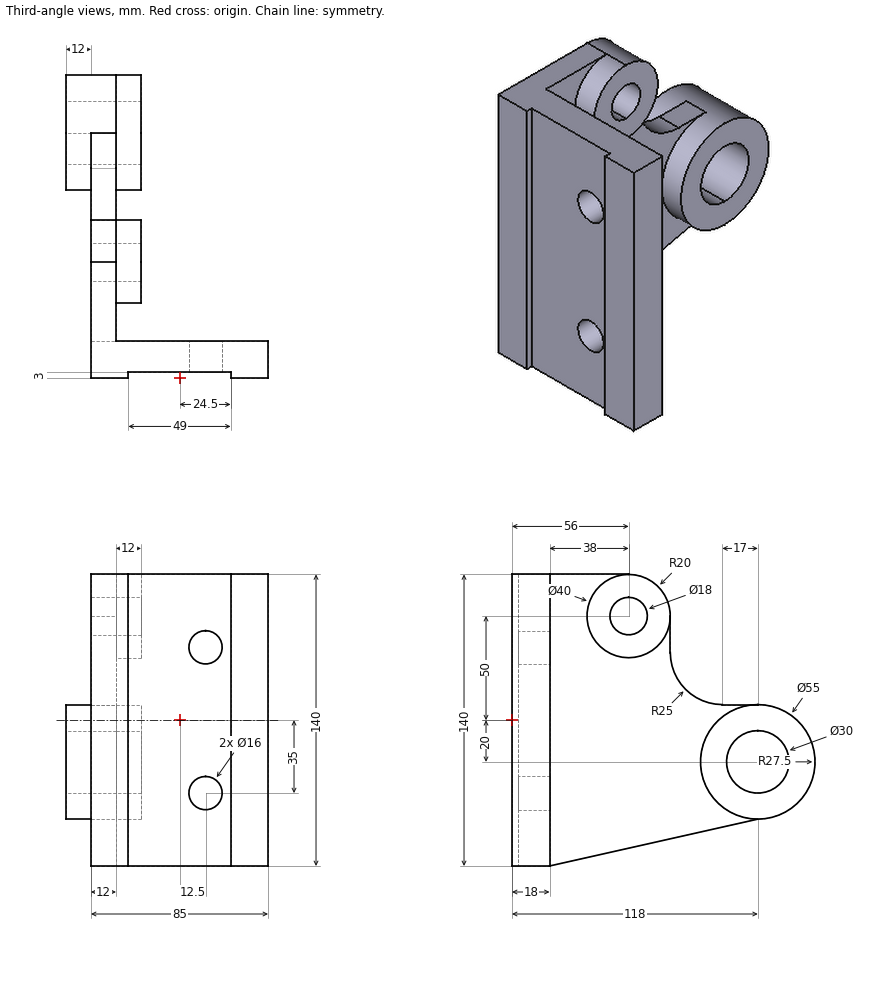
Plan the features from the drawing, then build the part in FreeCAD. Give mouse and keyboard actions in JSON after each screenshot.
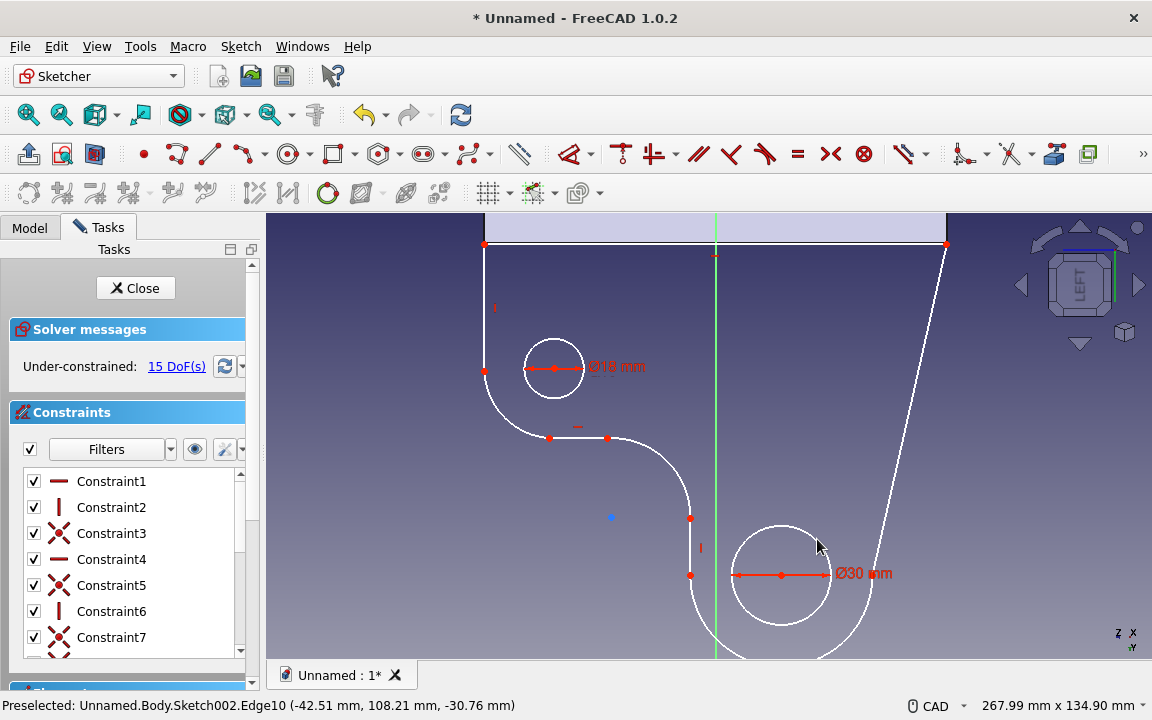
{"action": "left_click", "coordinate": [567, 438]}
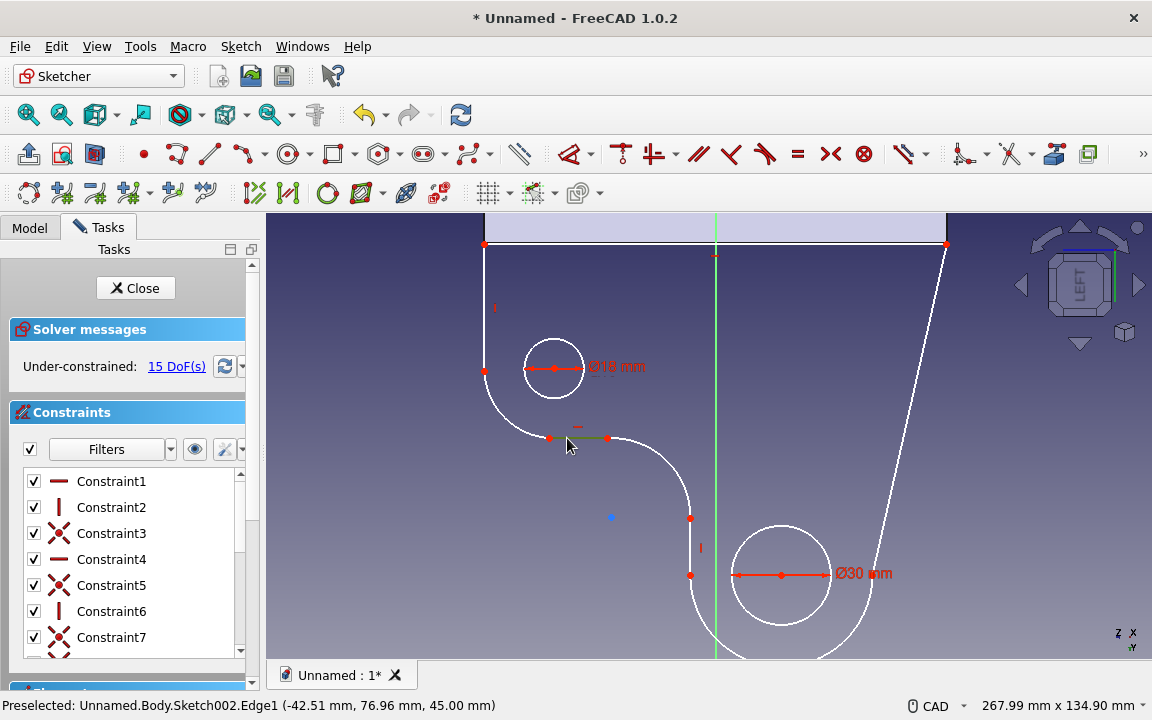
{"action": "left_click", "coordinate": [682, 481]}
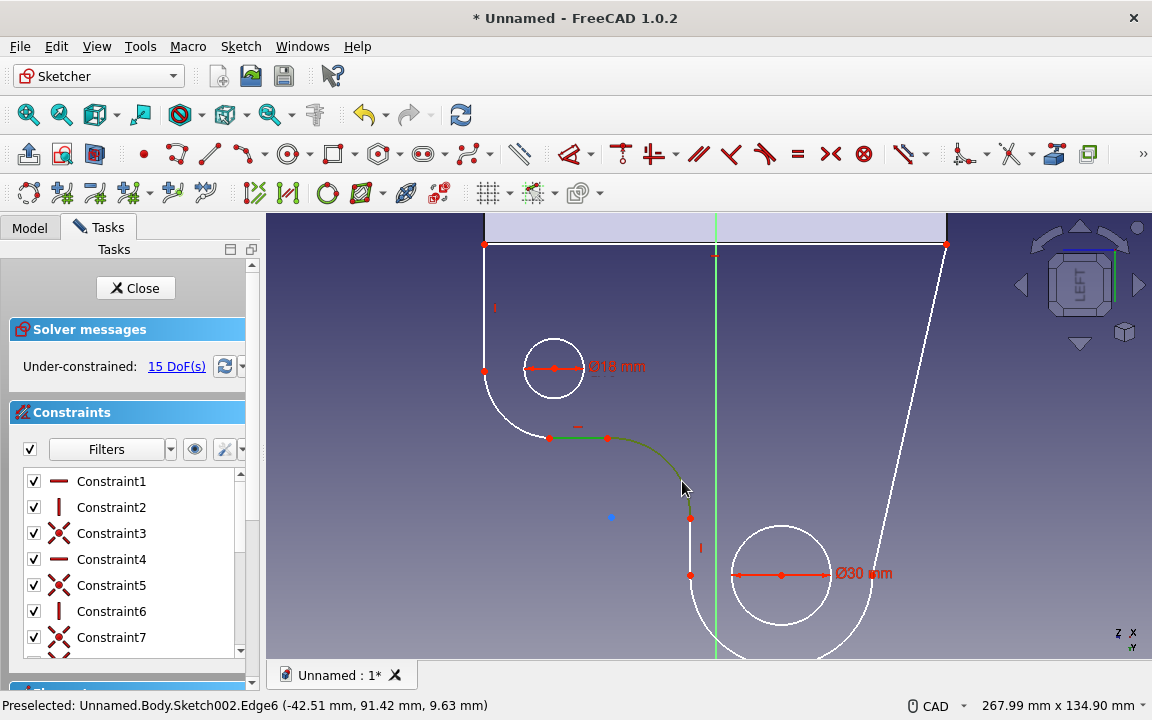
{"action": "key", "text": "t"}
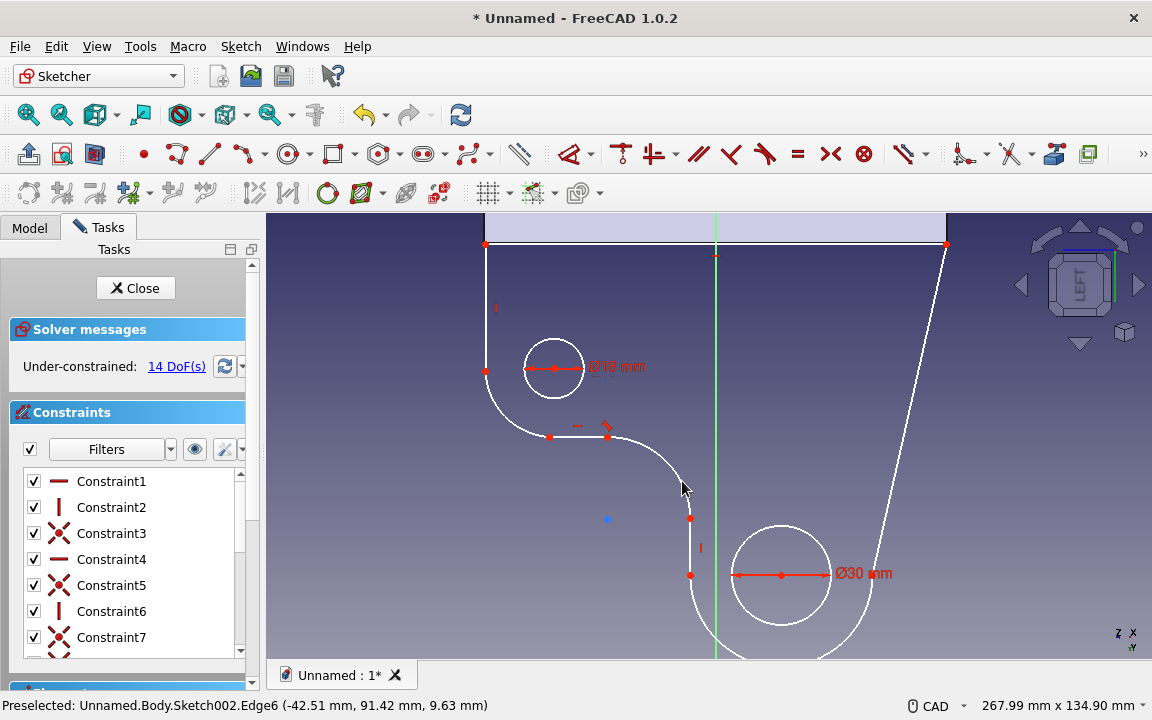
{"action": "left_click", "coordinate": [567, 437]}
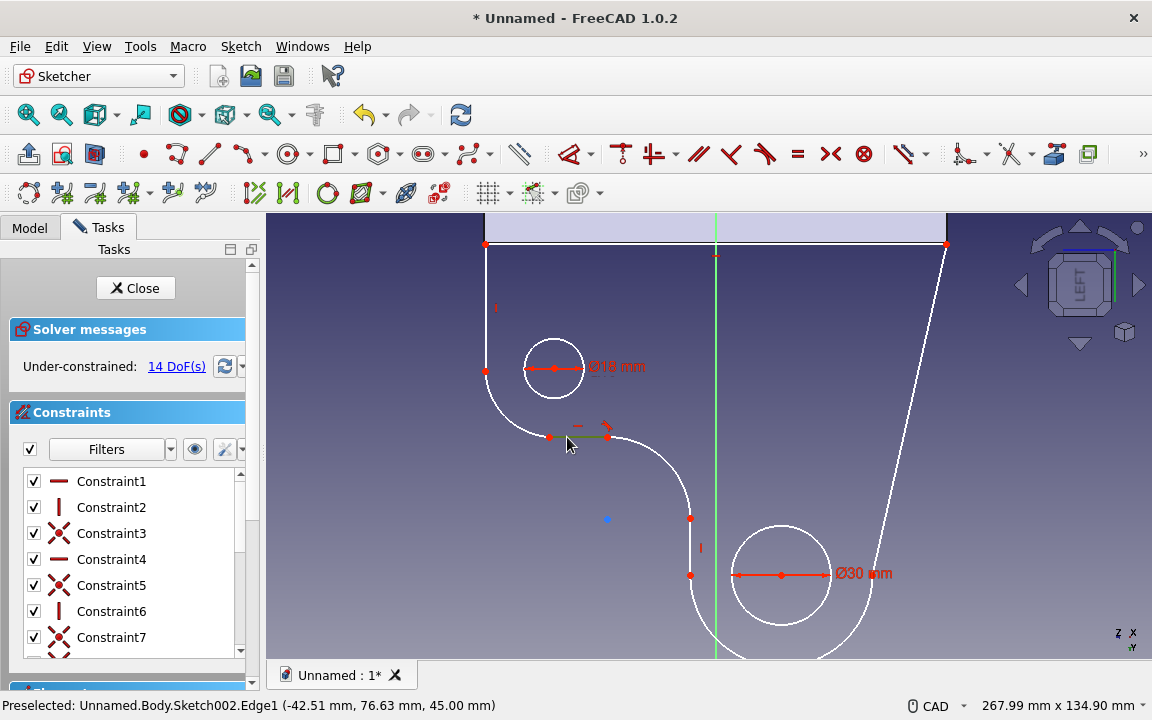
{"action": "left_click", "coordinate": [493, 400]}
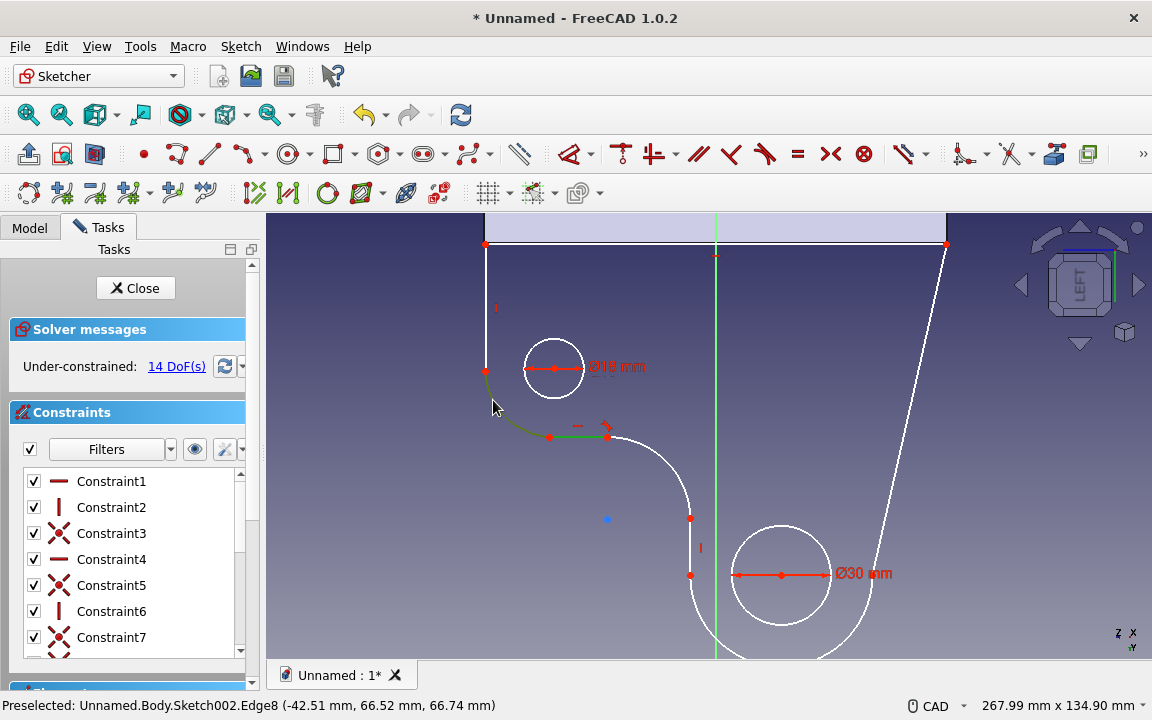
{"action": "key", "text": "t"}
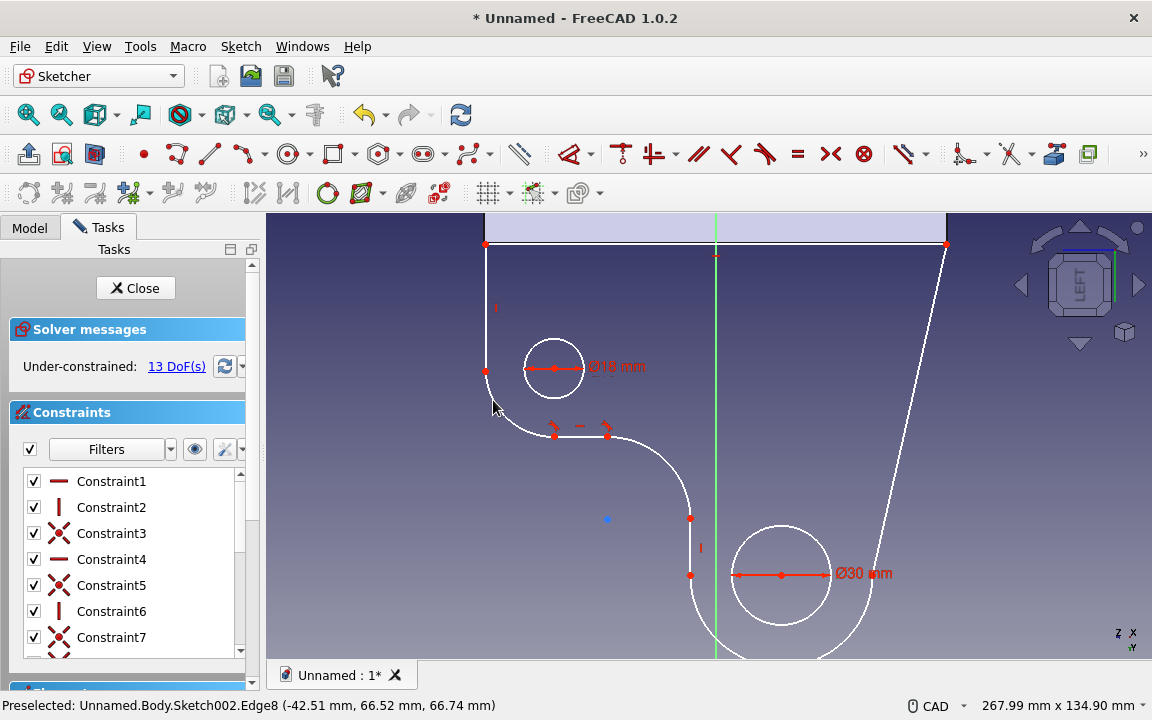
{"action": "left_click", "coordinate": [690, 536]}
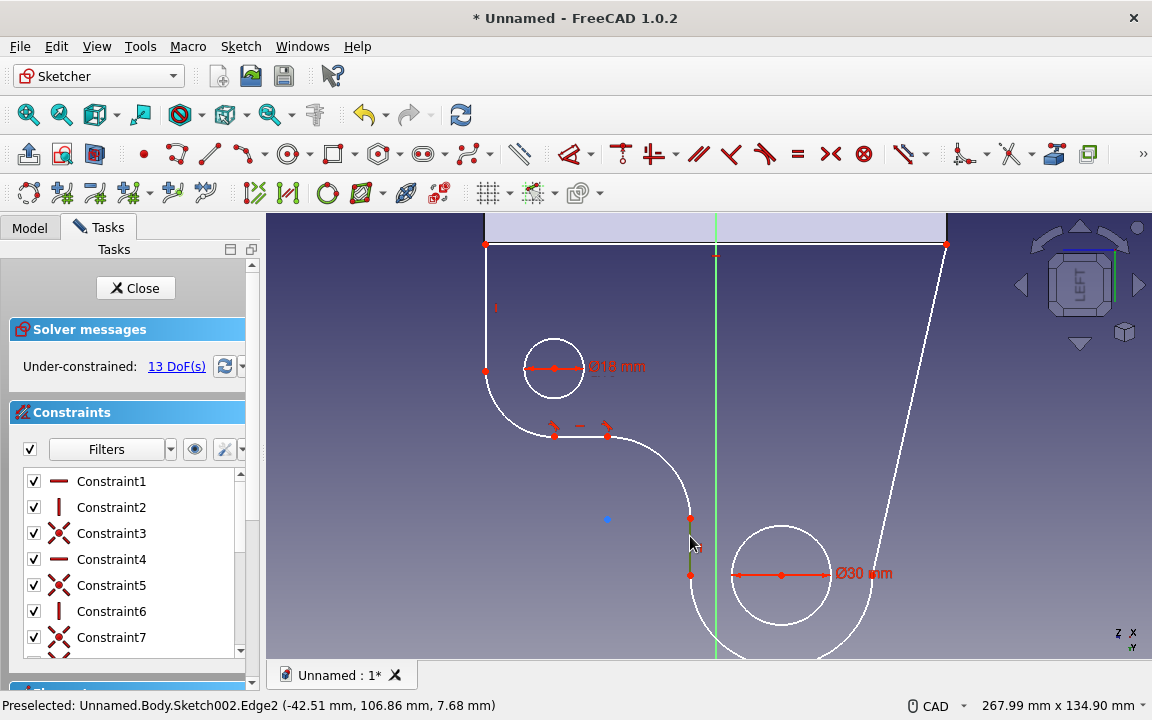
{"action": "left_click", "coordinate": [681, 482]}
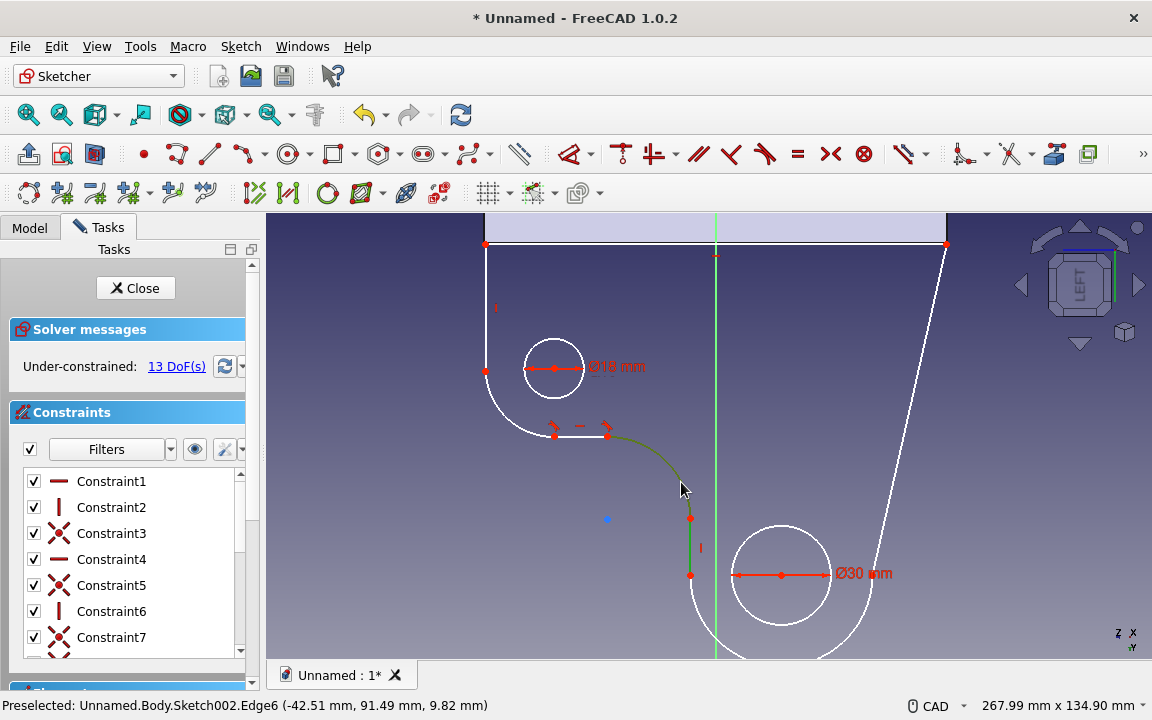
{"action": "key", "text": "t"}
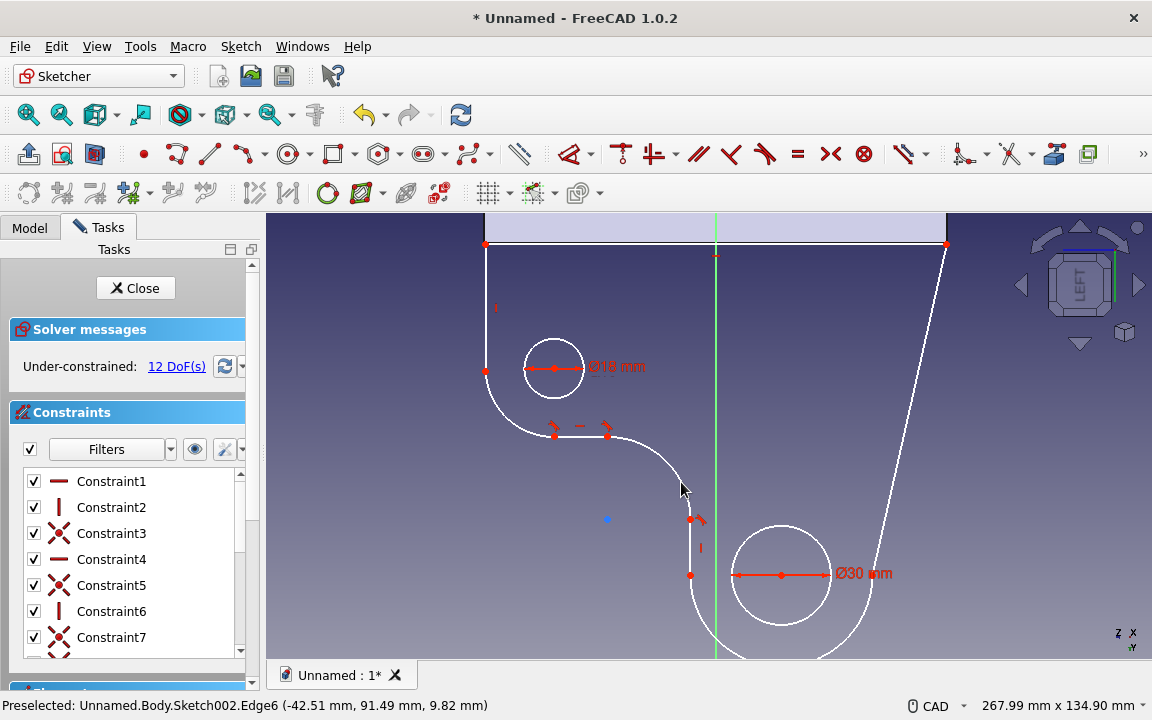
{"action": "left_click", "coordinate": [690, 536]}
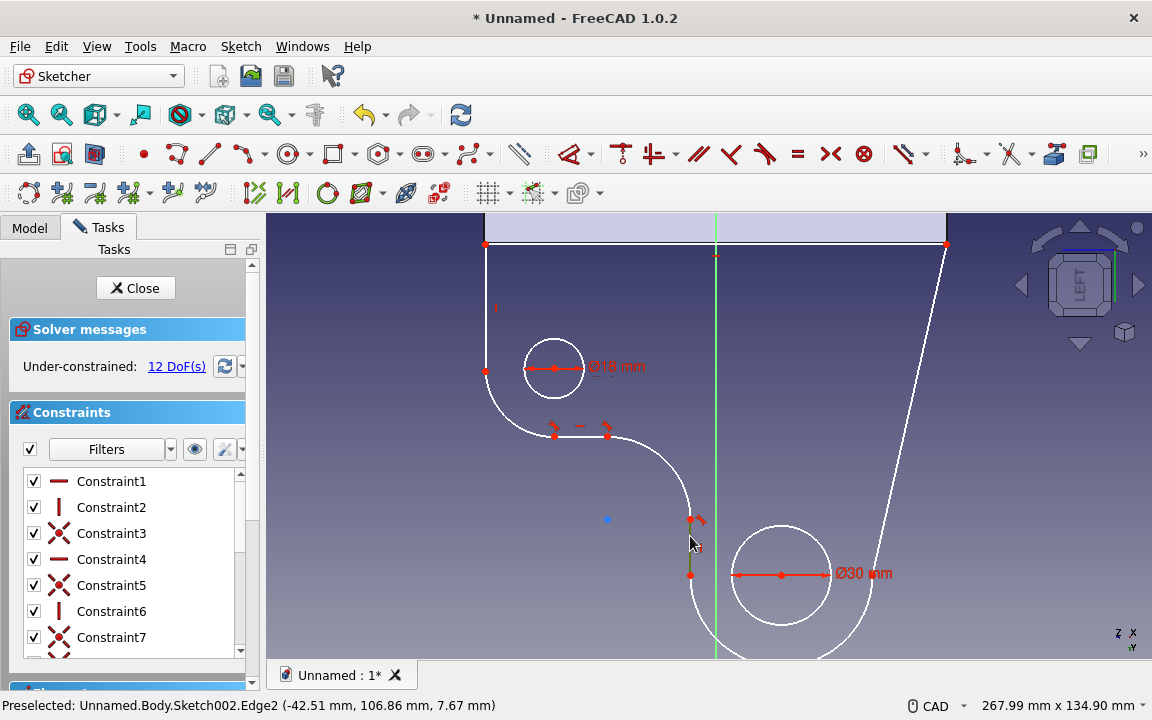
{"action": "left_click", "coordinate": [855, 629]}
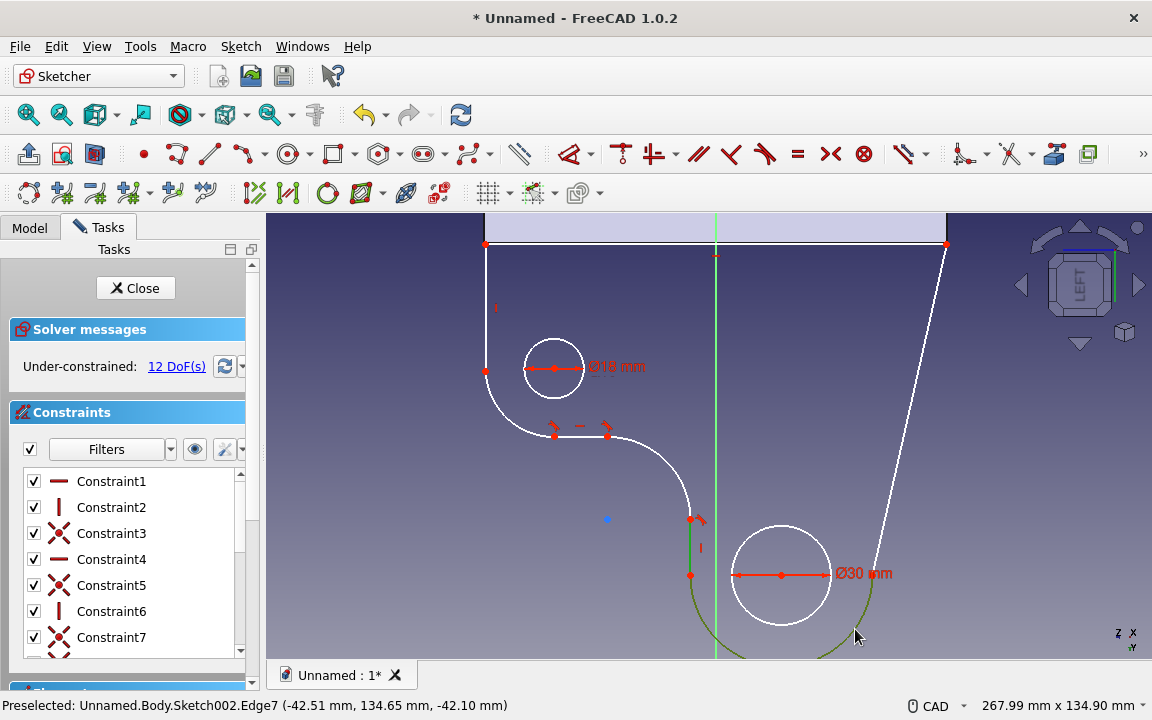
{"action": "left_click", "coordinate": [765, 154]}